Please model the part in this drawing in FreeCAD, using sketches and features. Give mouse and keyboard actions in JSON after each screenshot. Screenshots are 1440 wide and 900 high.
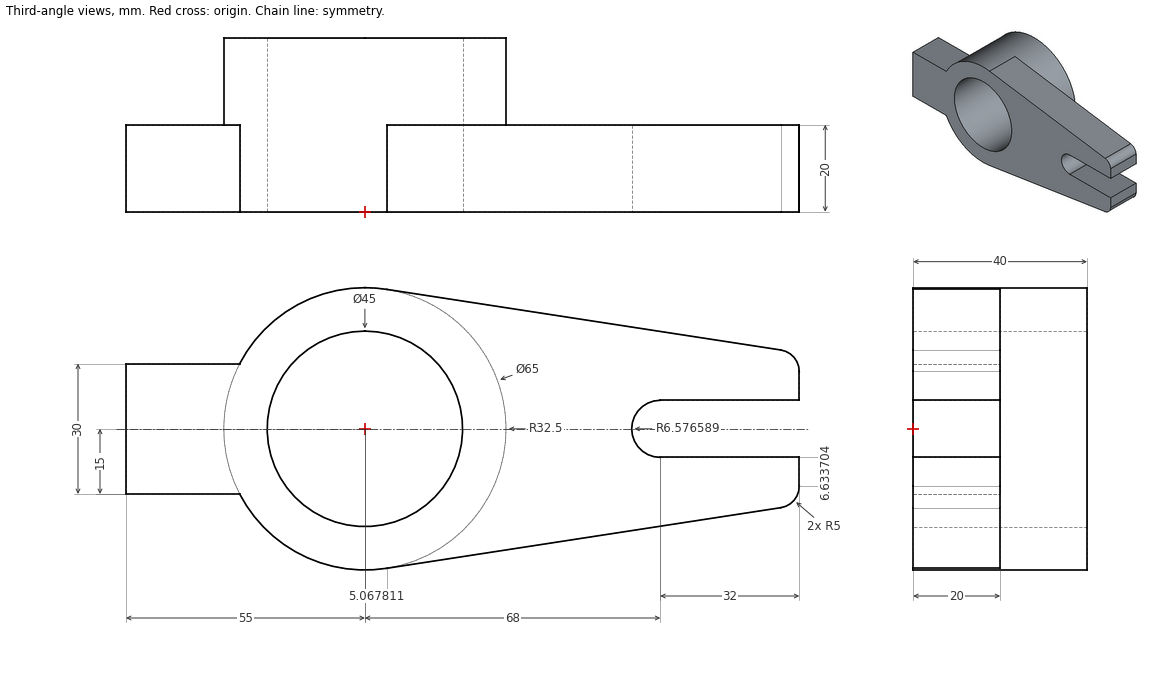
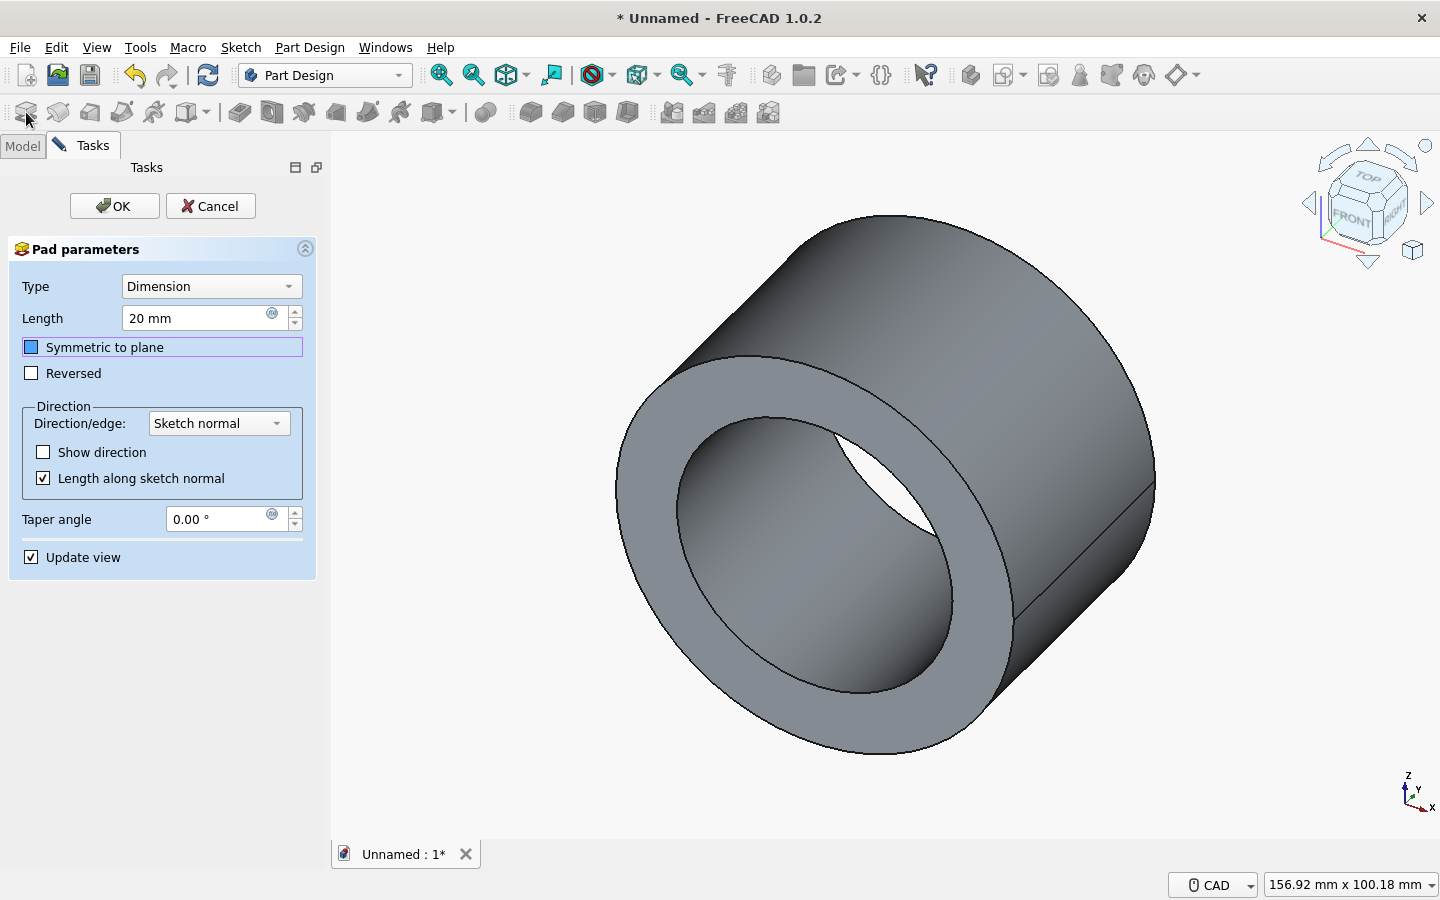
{"action": "left_click", "coordinate": [30, 373]}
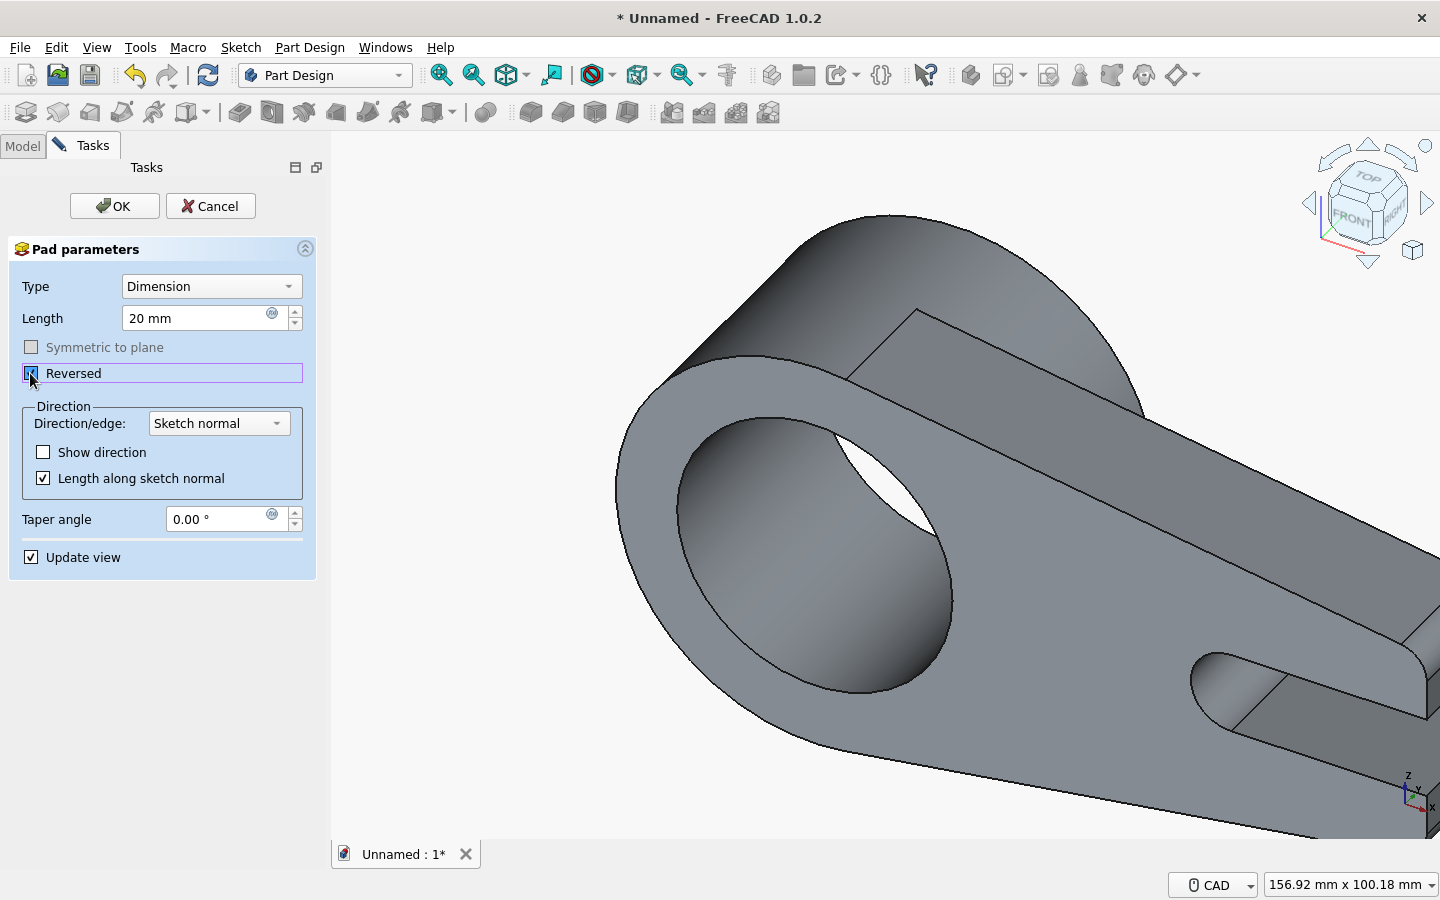
{"action": "left_click", "coordinate": [115, 206]}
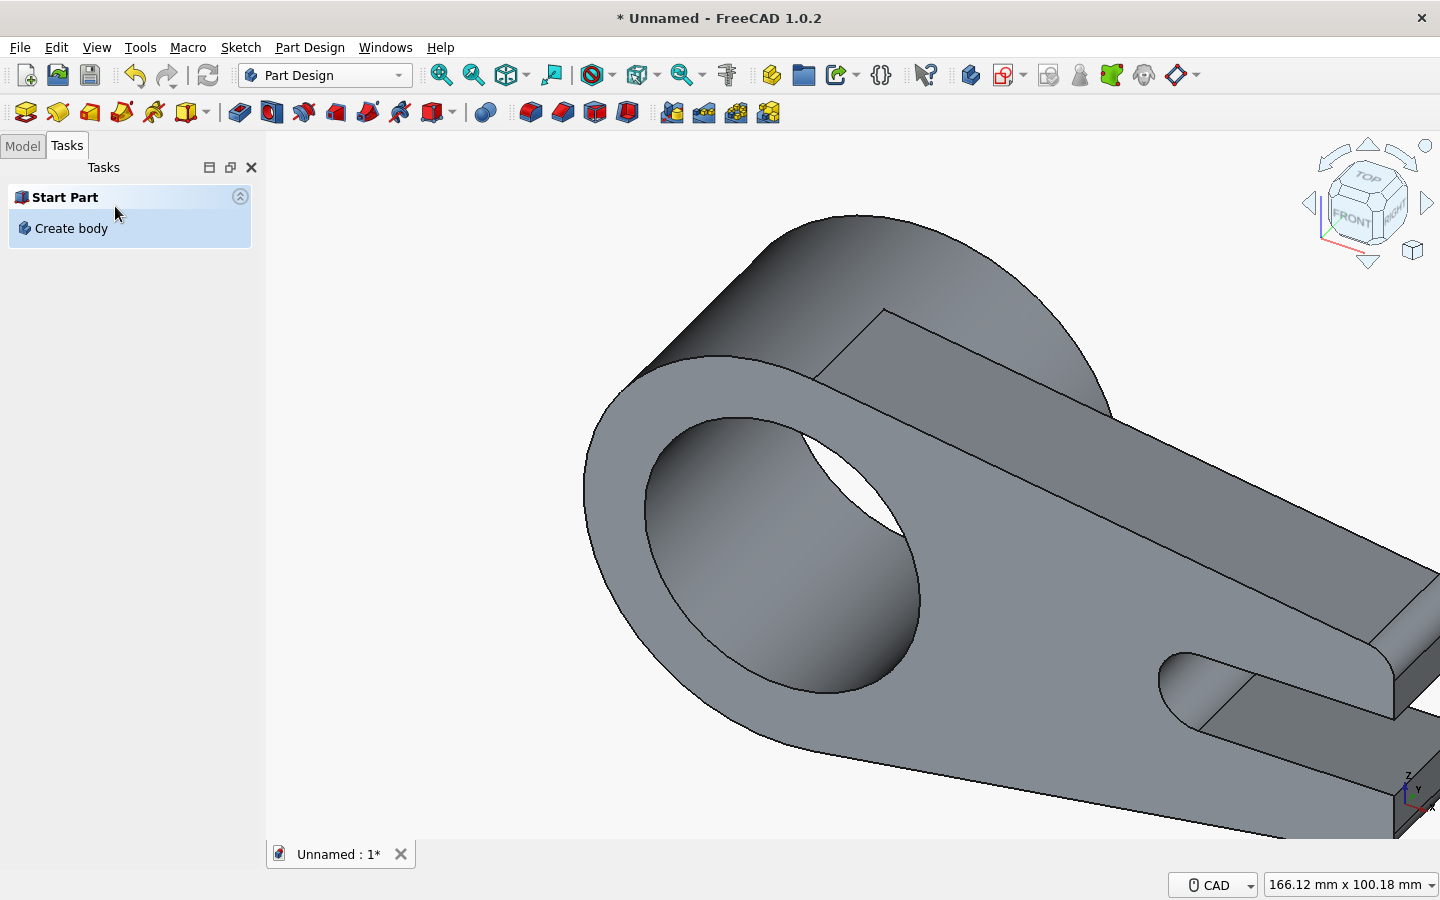
{"action": "left_click", "coordinate": [442, 76]}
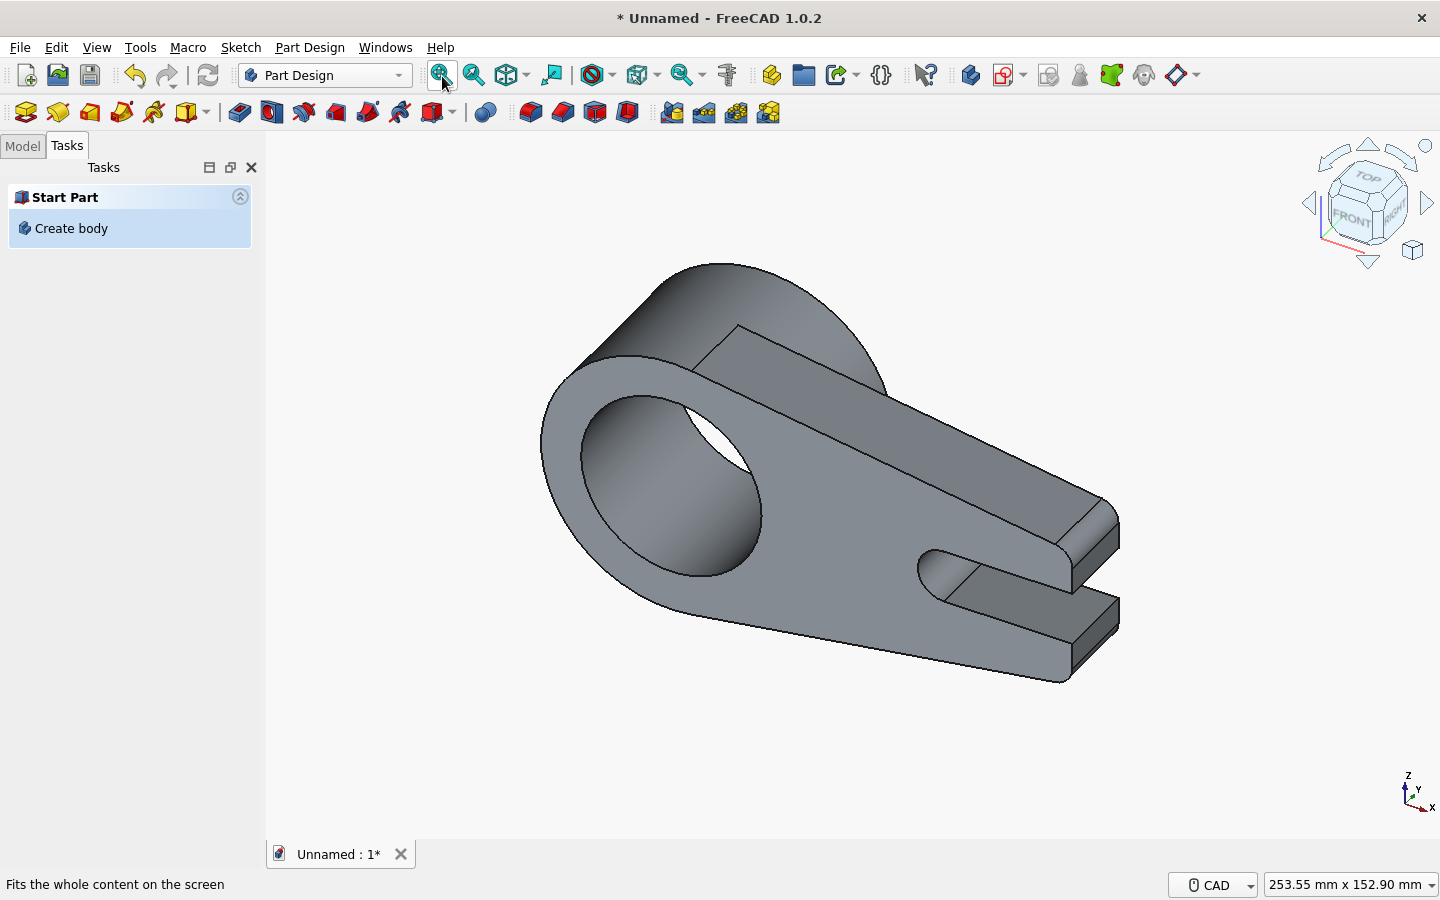
{"action": "left_click", "coordinate": [807, 495]}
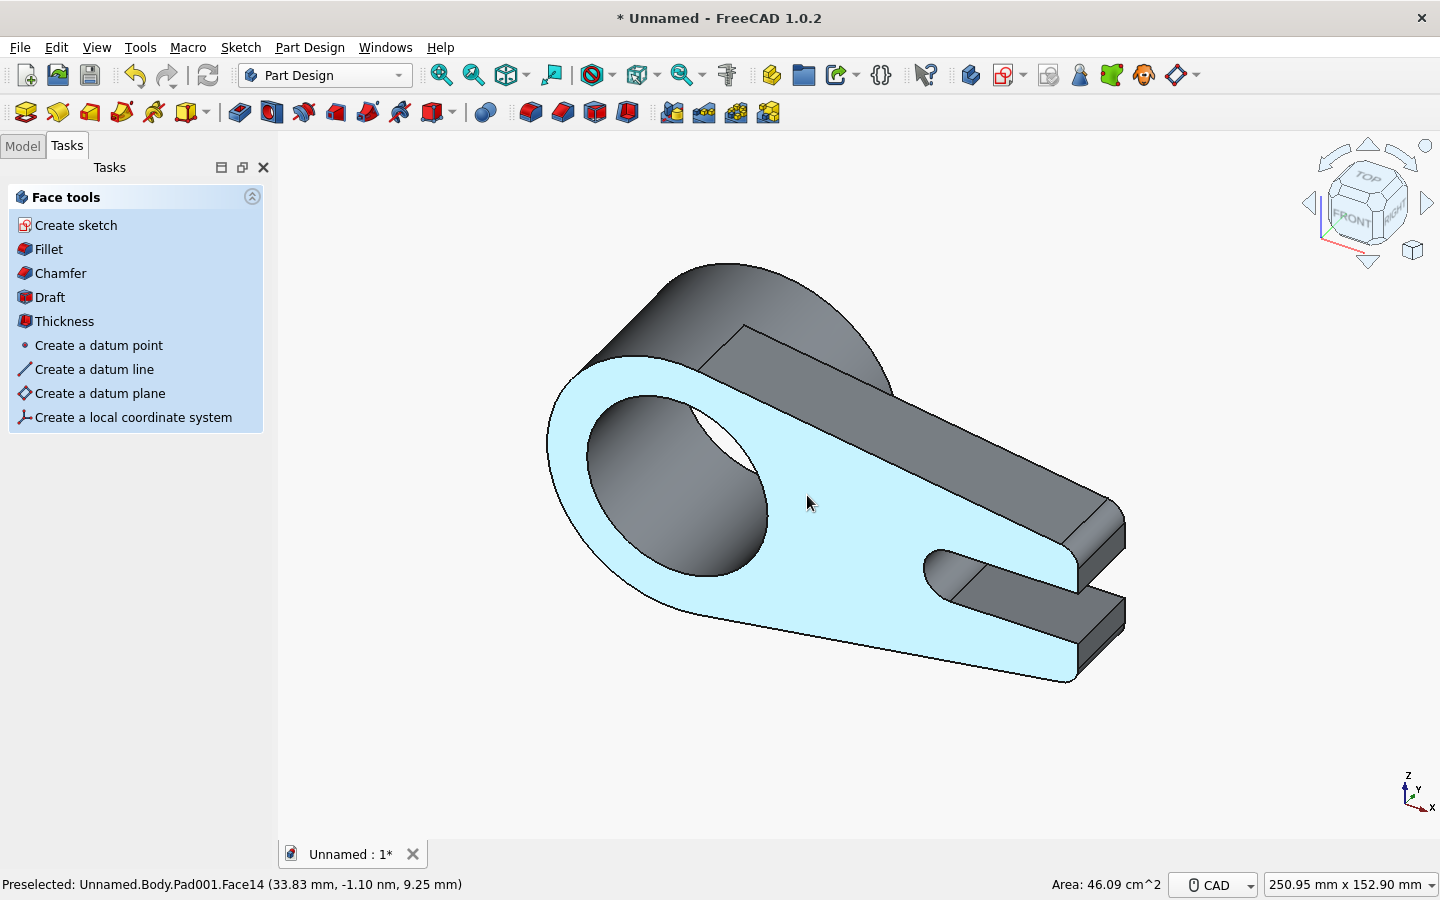
{"action": "left_click", "coordinate": [1004, 76]}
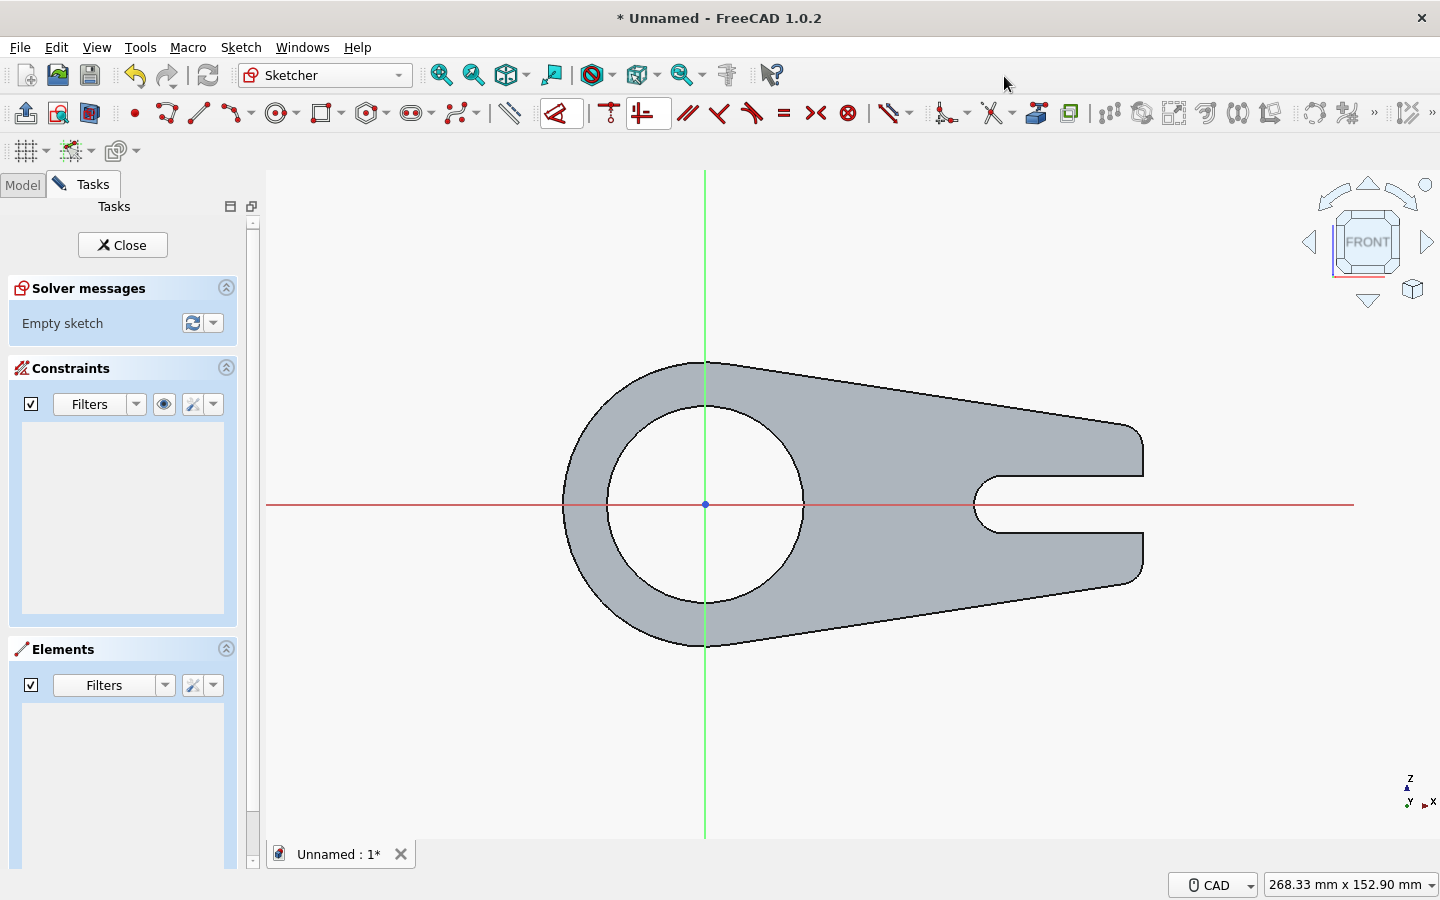
{"action": "scroll", "coordinate": [469, 505], "scroll_direction": "up", "scroll_amount": 5}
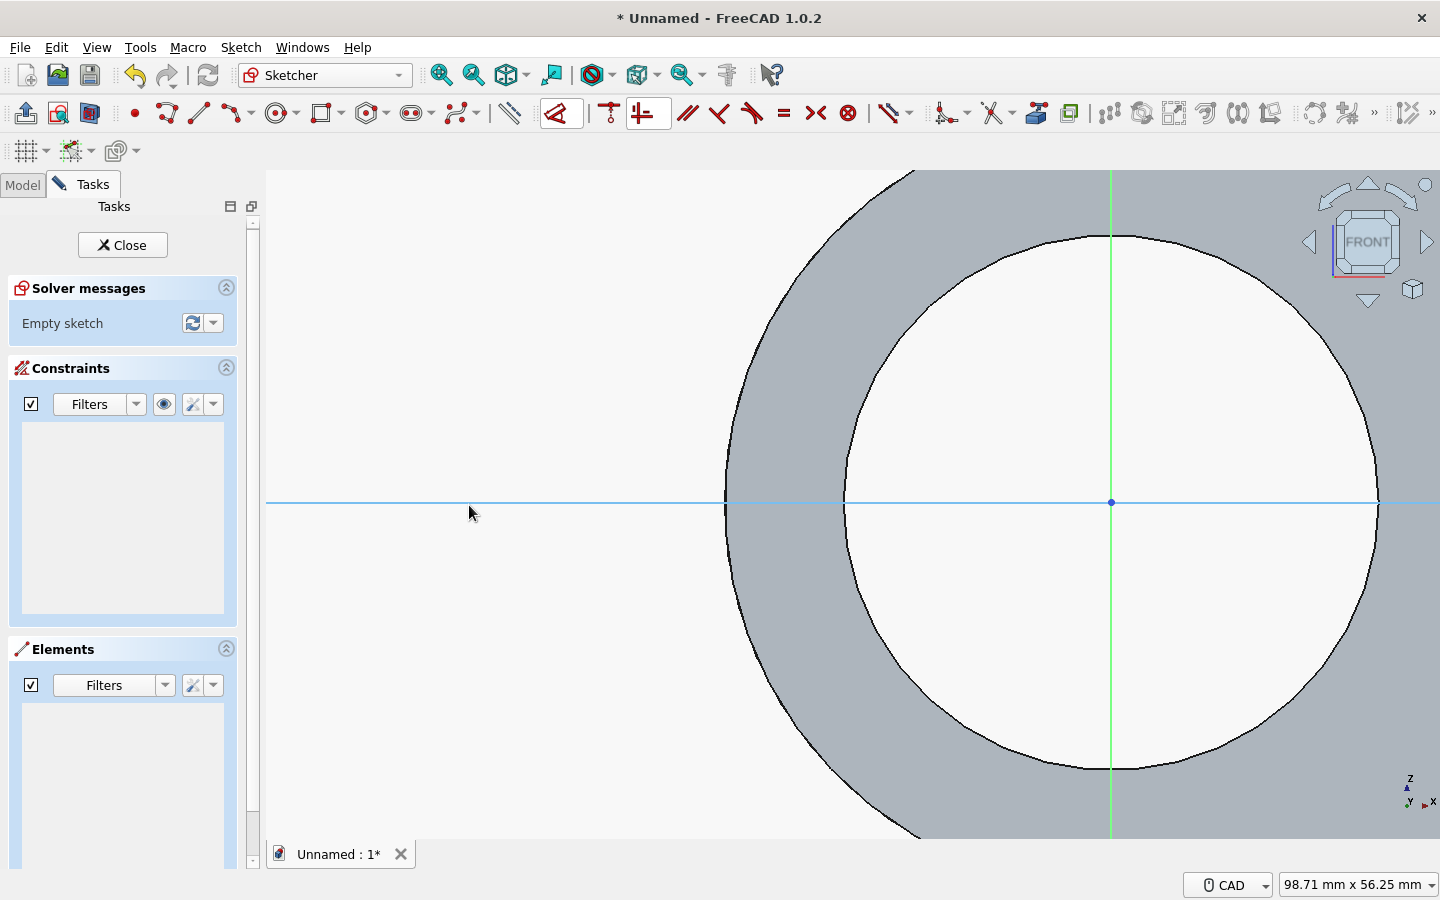
{"action": "left_click", "coordinate": [168, 114]}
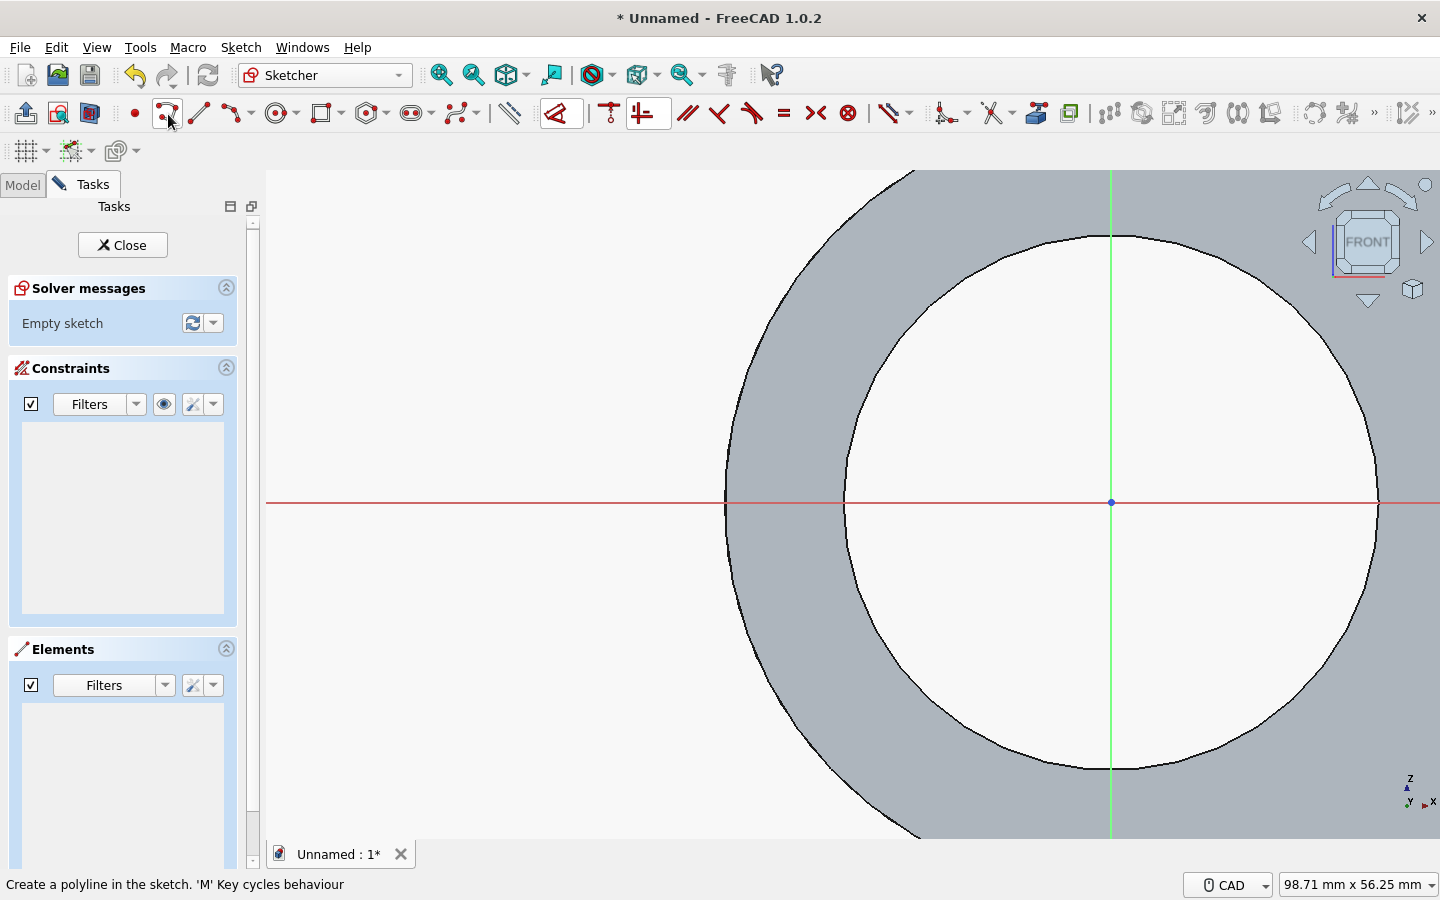
{"action": "left_click", "coordinate": [768, 681]}
{"action": "left_click", "coordinate": [457, 681]}
{"action": "left_click", "coordinate": [457, 324]}
{"action": "left_click", "coordinate": [768, 324]}
{"action": "right_click", "coordinate": [768, 324]}